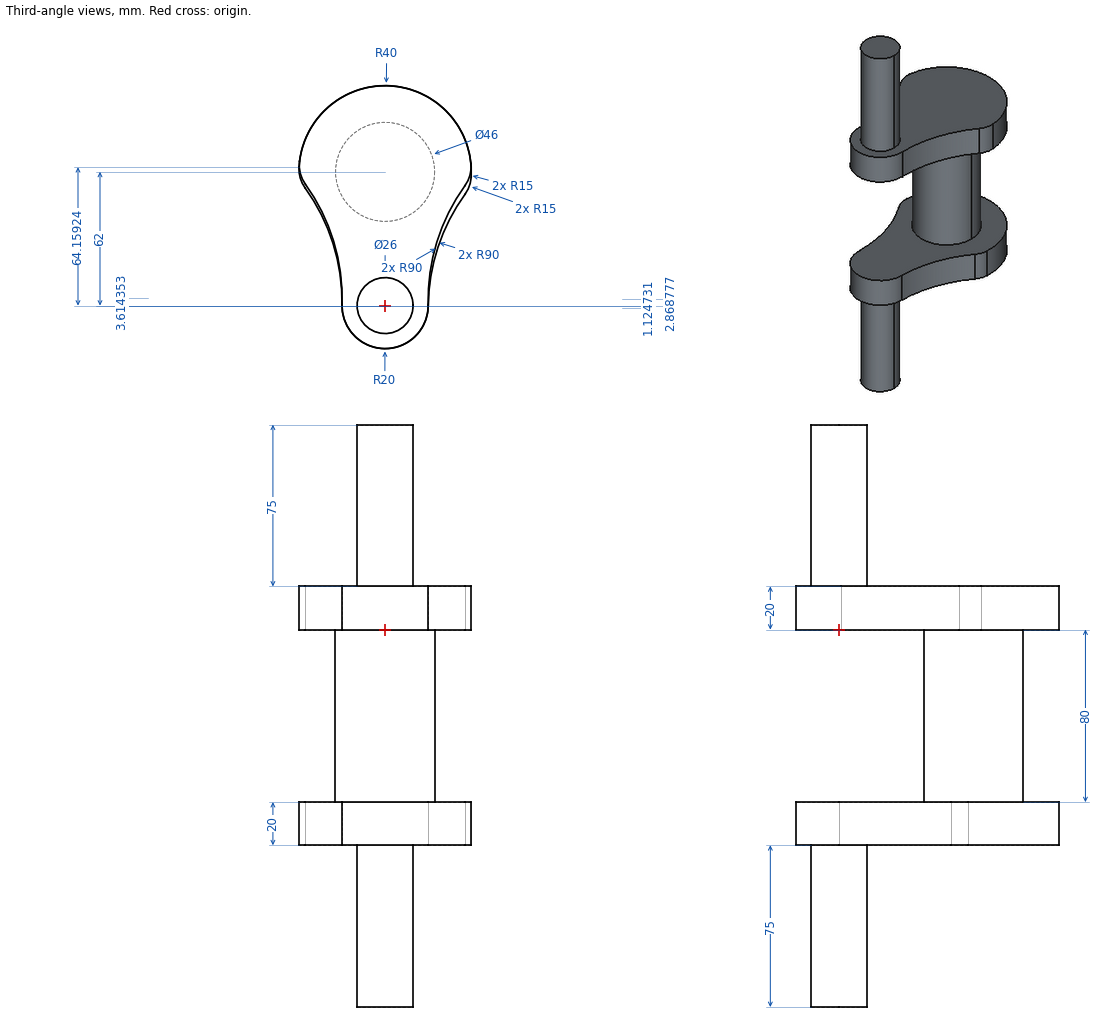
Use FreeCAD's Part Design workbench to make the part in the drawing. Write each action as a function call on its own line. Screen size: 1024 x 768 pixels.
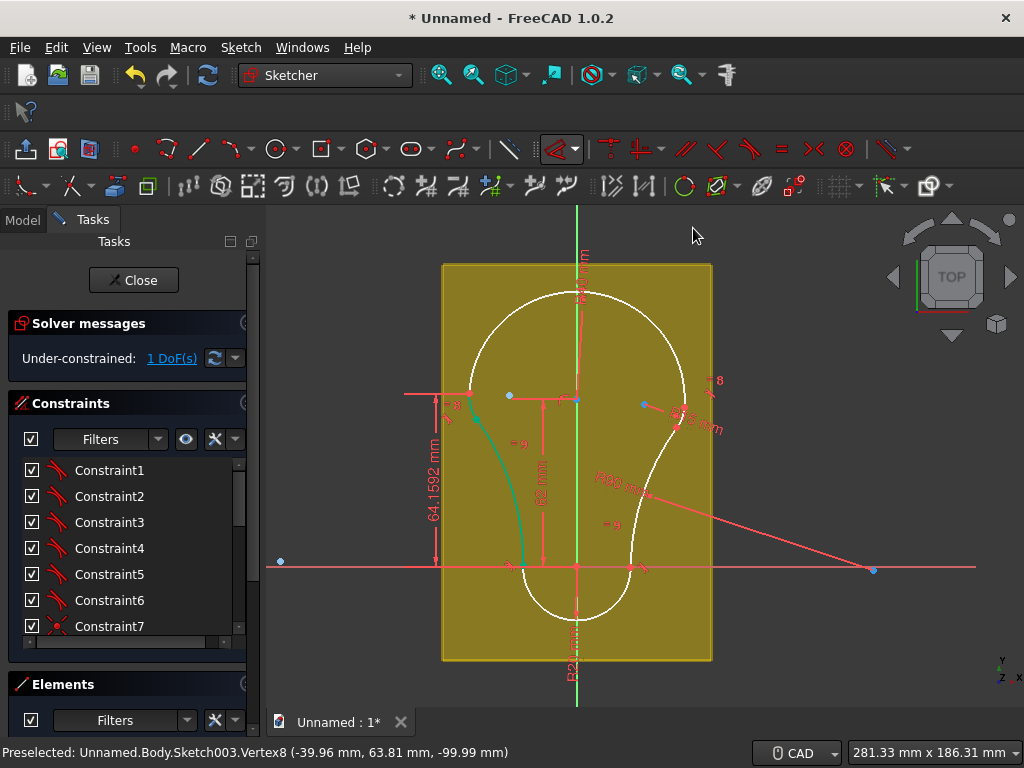
scroll(294, 455, down, 1)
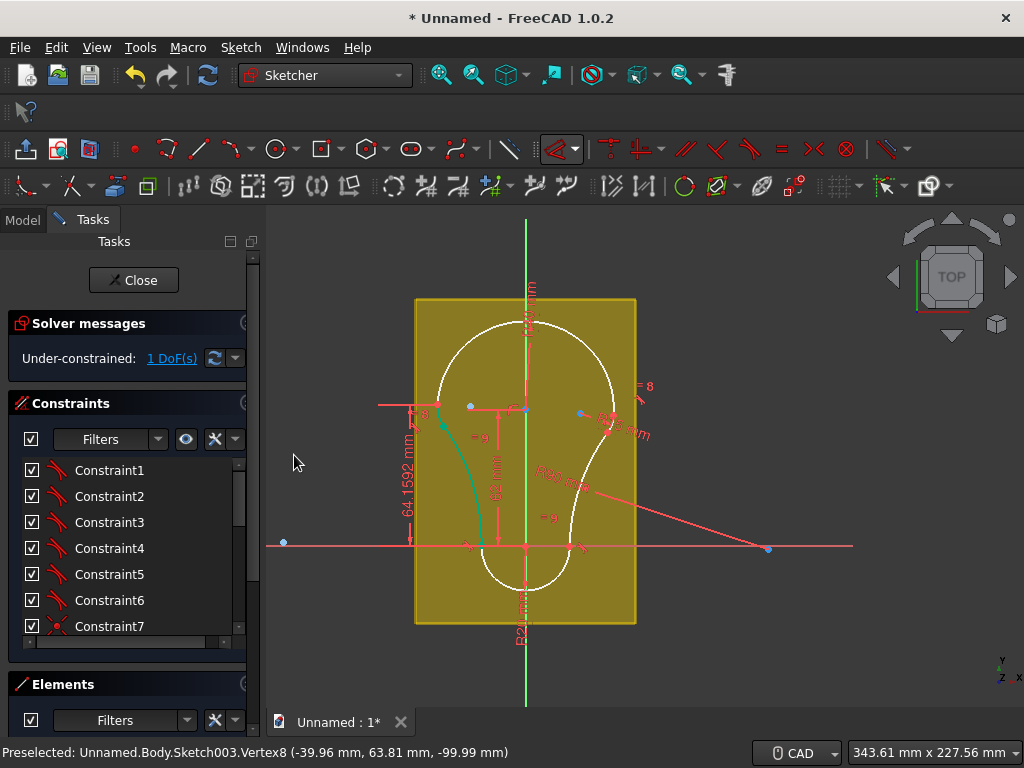
scroll(768, 549, up, 14)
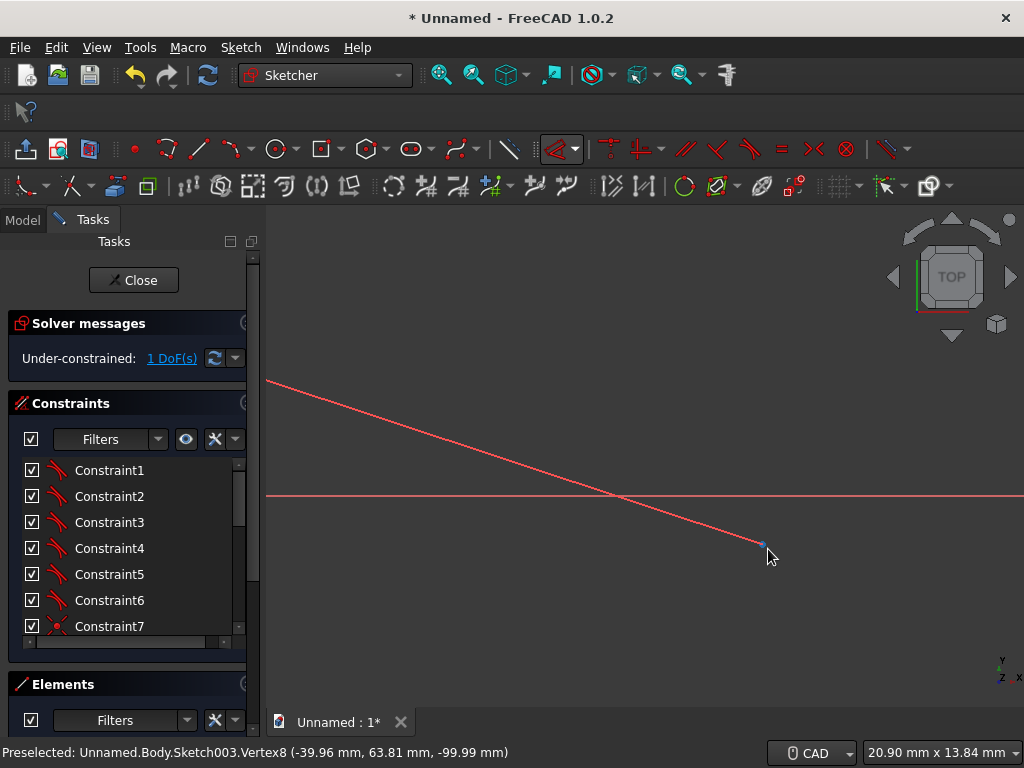
click(762, 544)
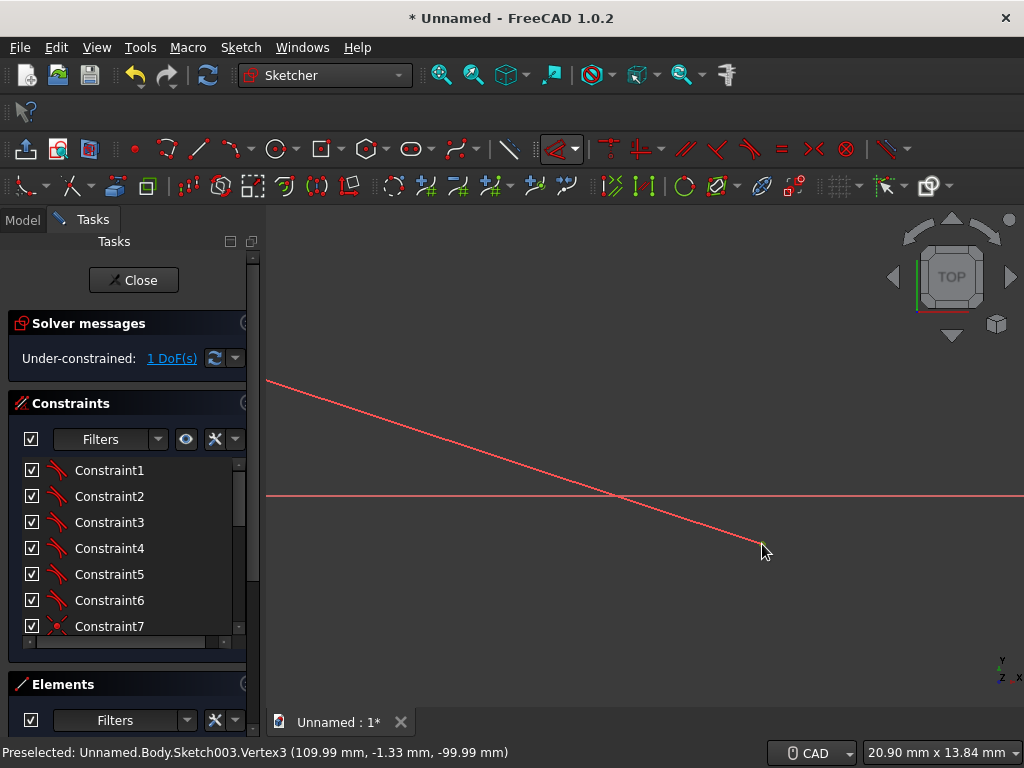
click(578, 150)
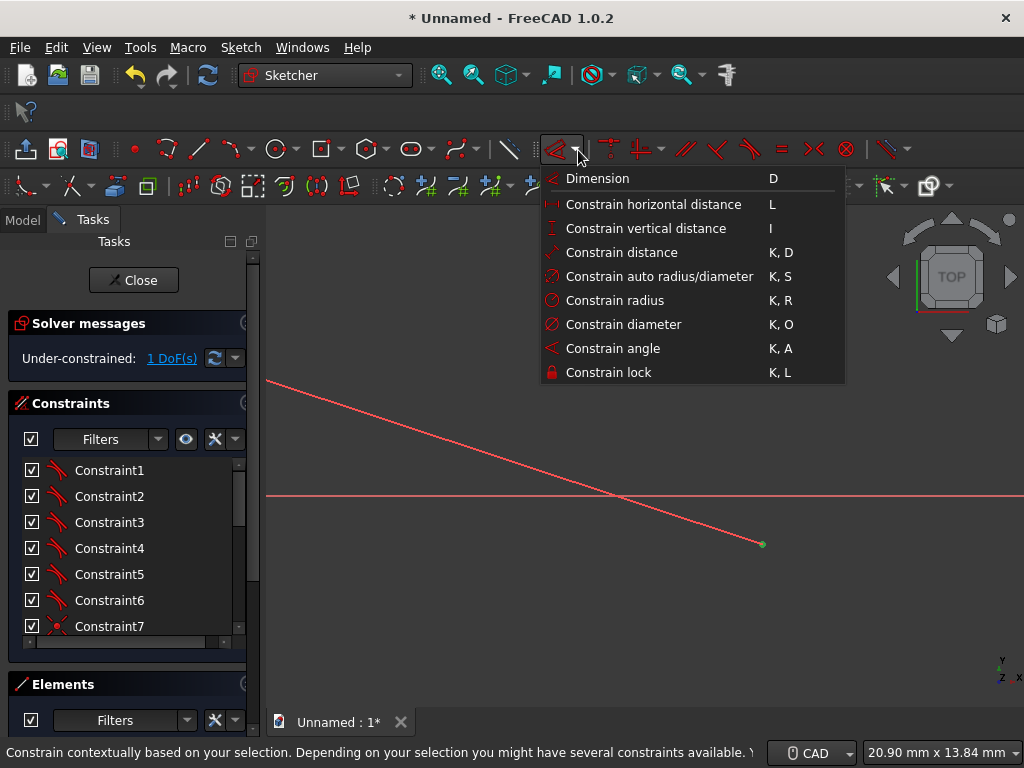
click(693, 228)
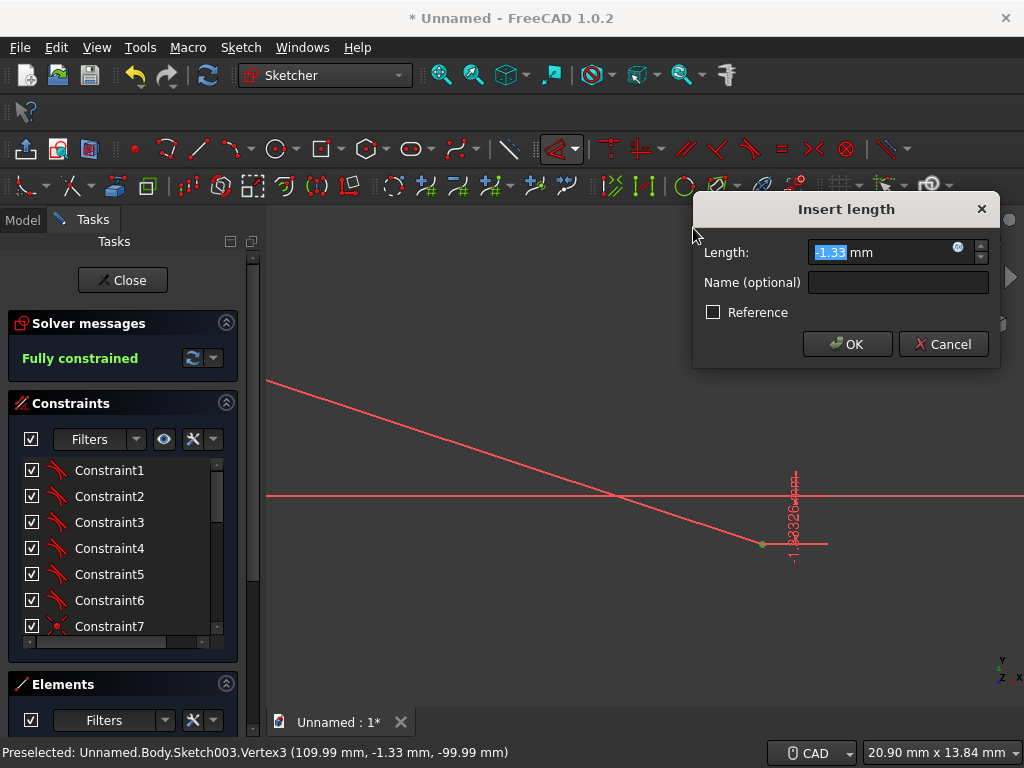
text(-1.124731)
key(Return)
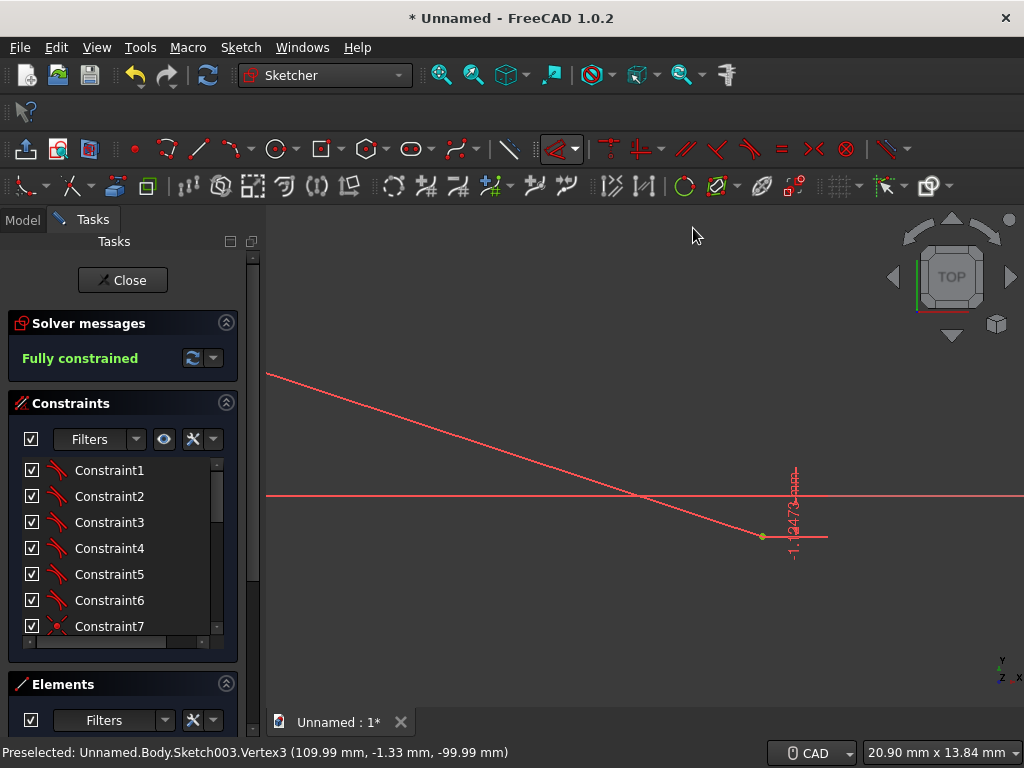
click(123, 280)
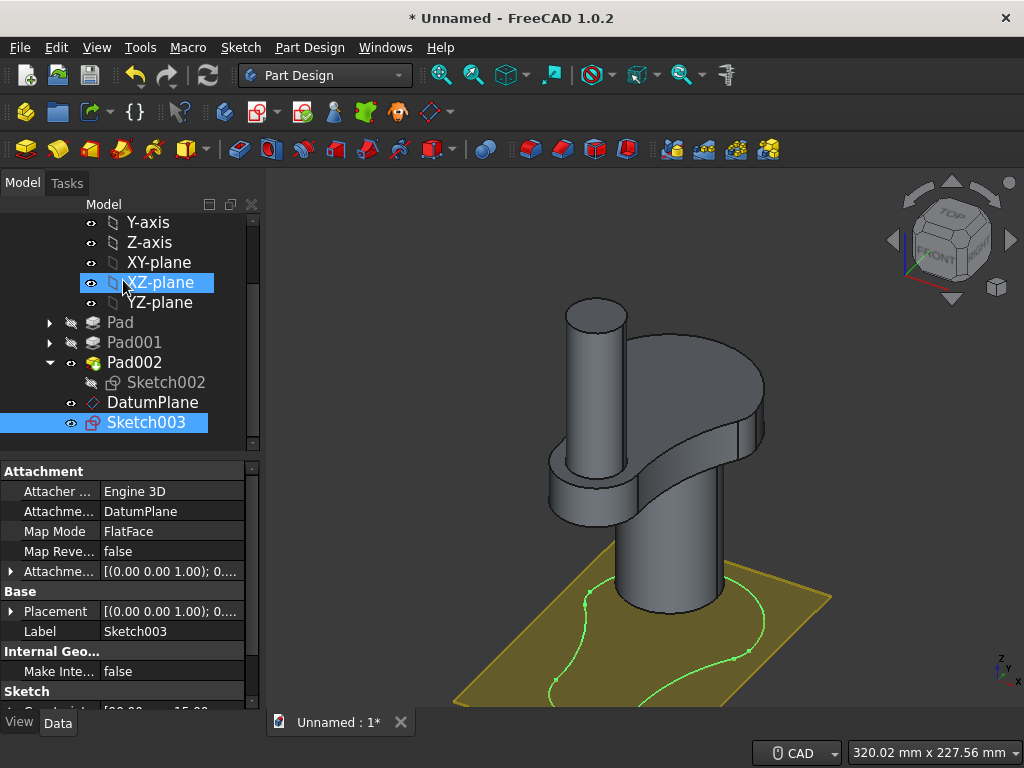
click(26, 150)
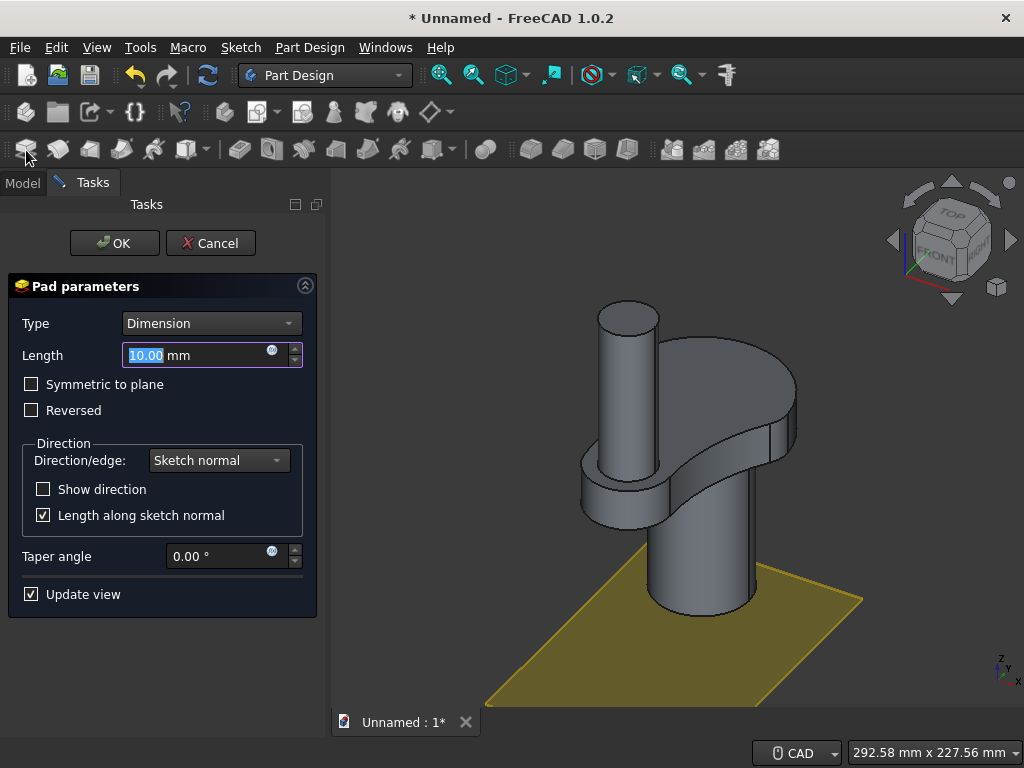
text(20)
key(Tab)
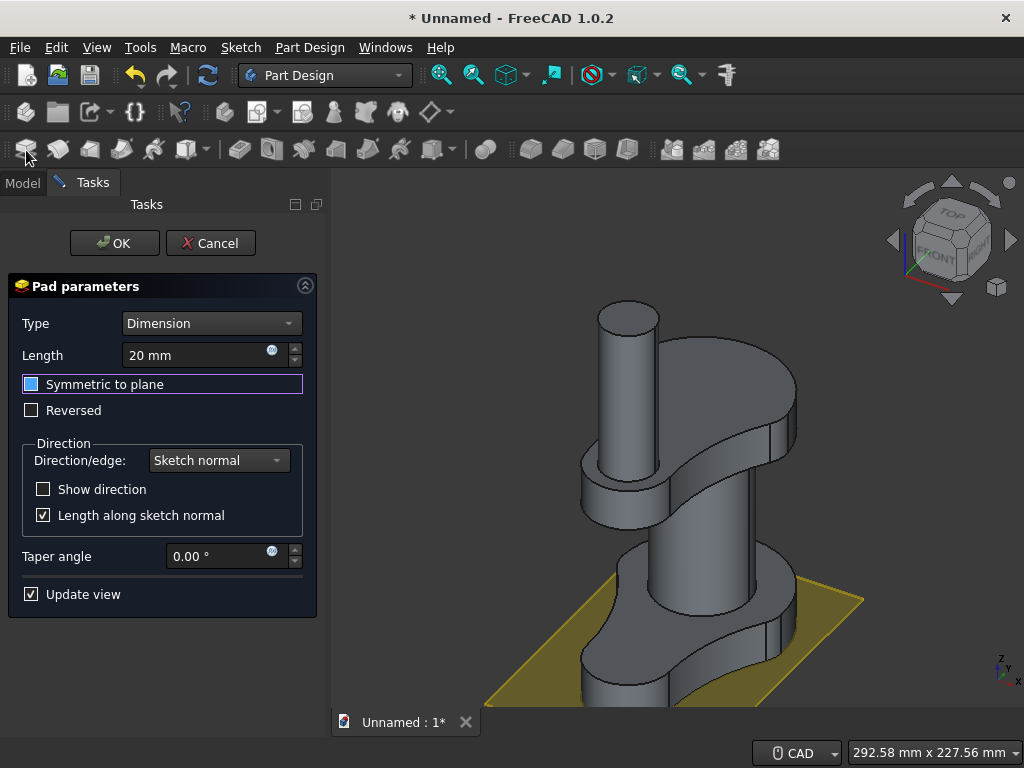
click(115, 243)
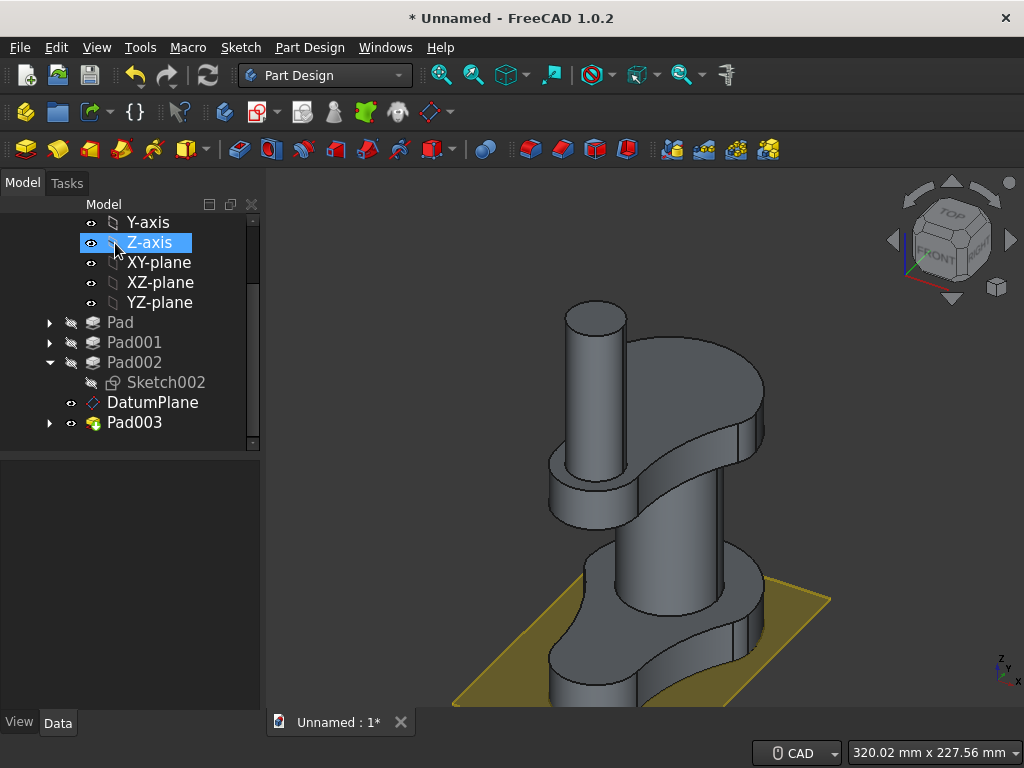
click(116, 403)
key(space)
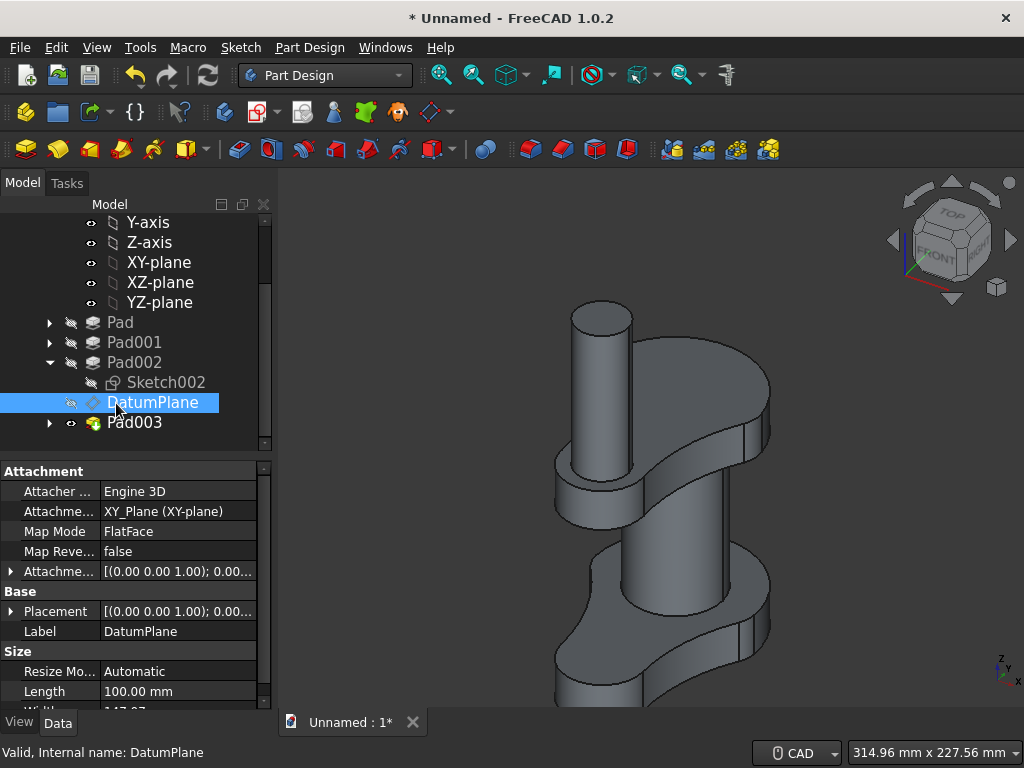
click(442, 76)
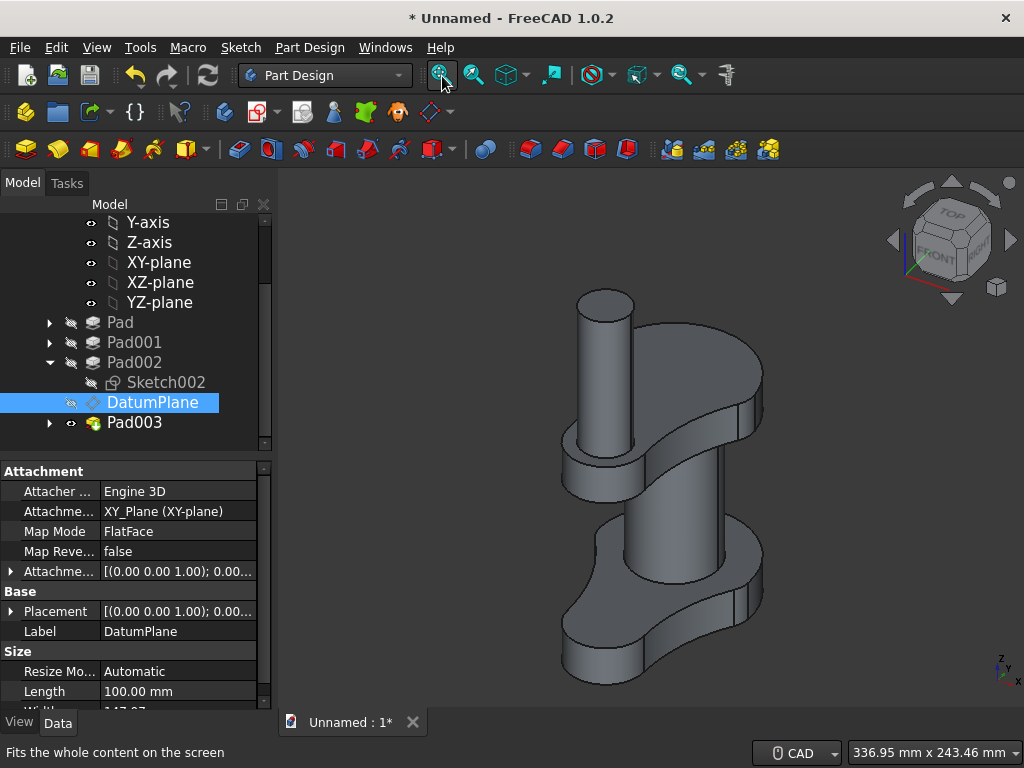
scroll(160, 318, down, 3)